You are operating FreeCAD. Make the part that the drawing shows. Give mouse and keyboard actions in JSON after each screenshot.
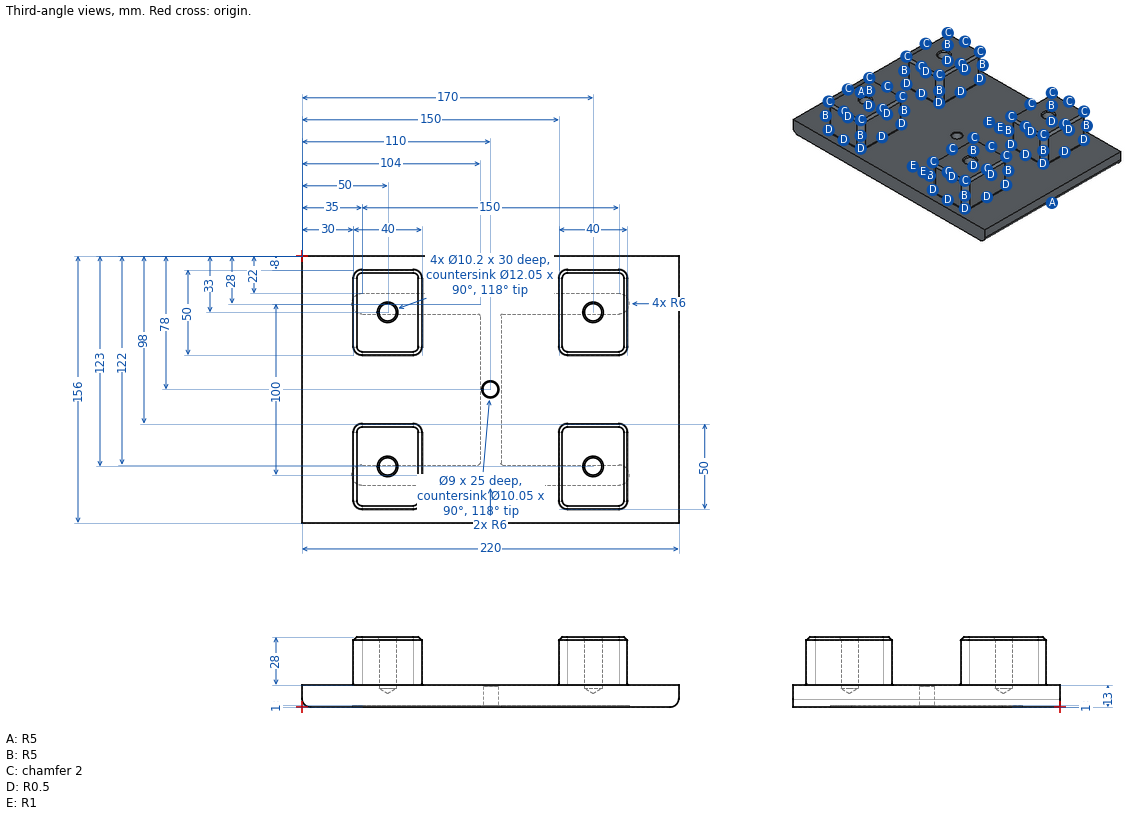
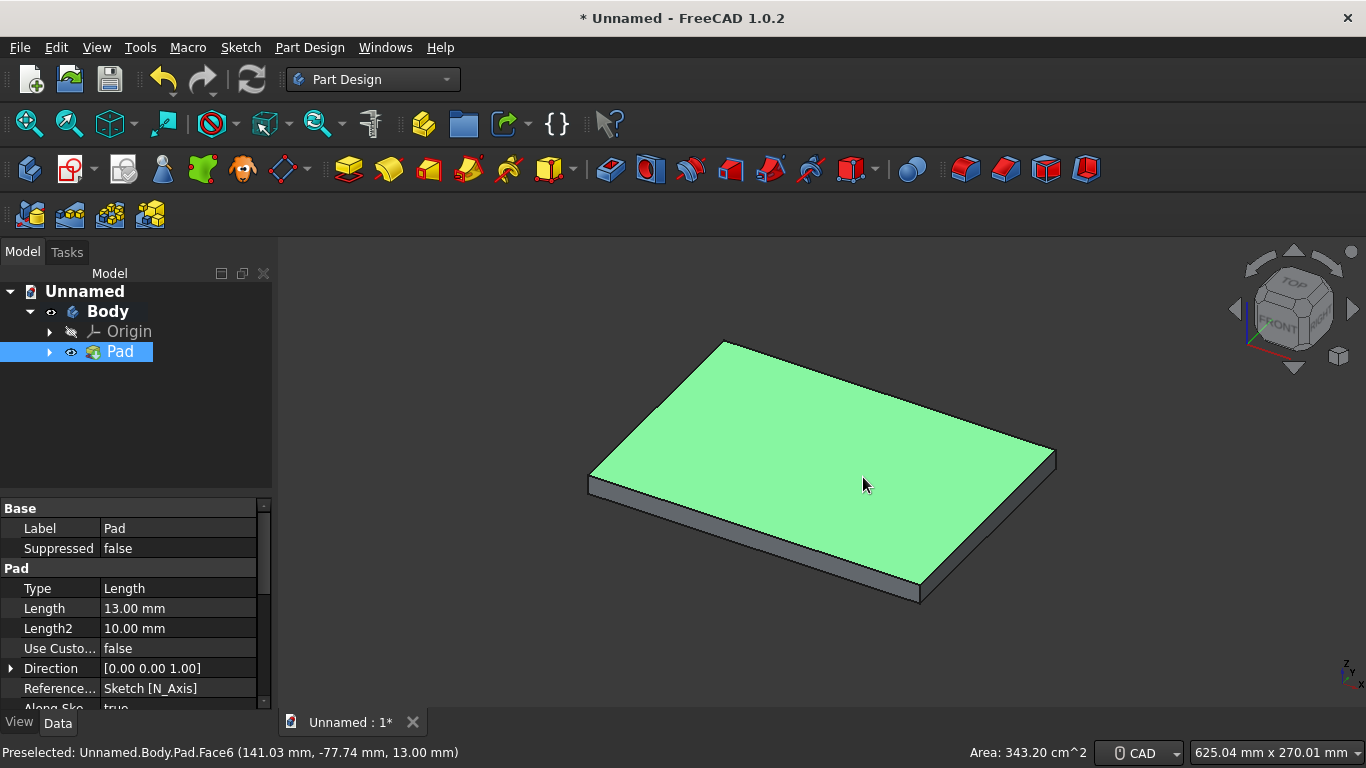
{"action": "left_click", "coordinate": [70, 170]}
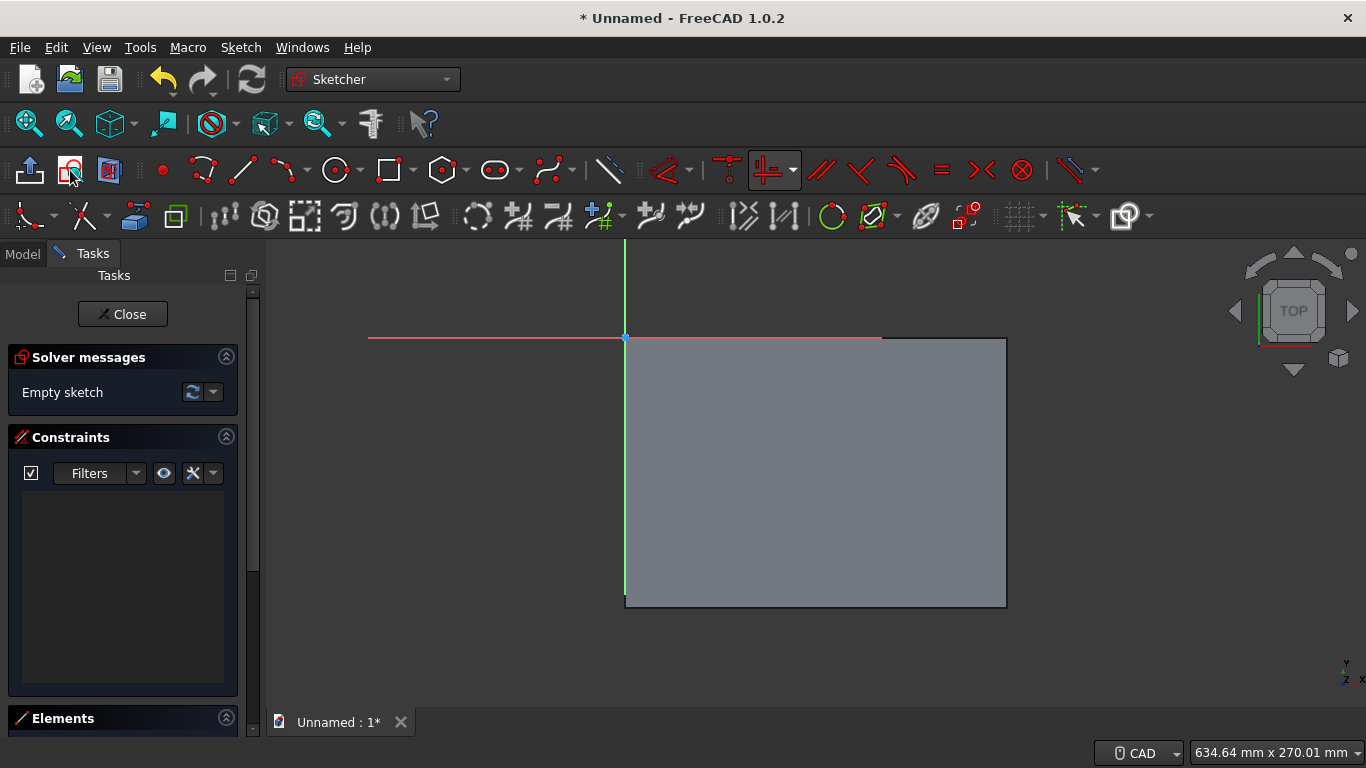
{"action": "key", "text": "g r"}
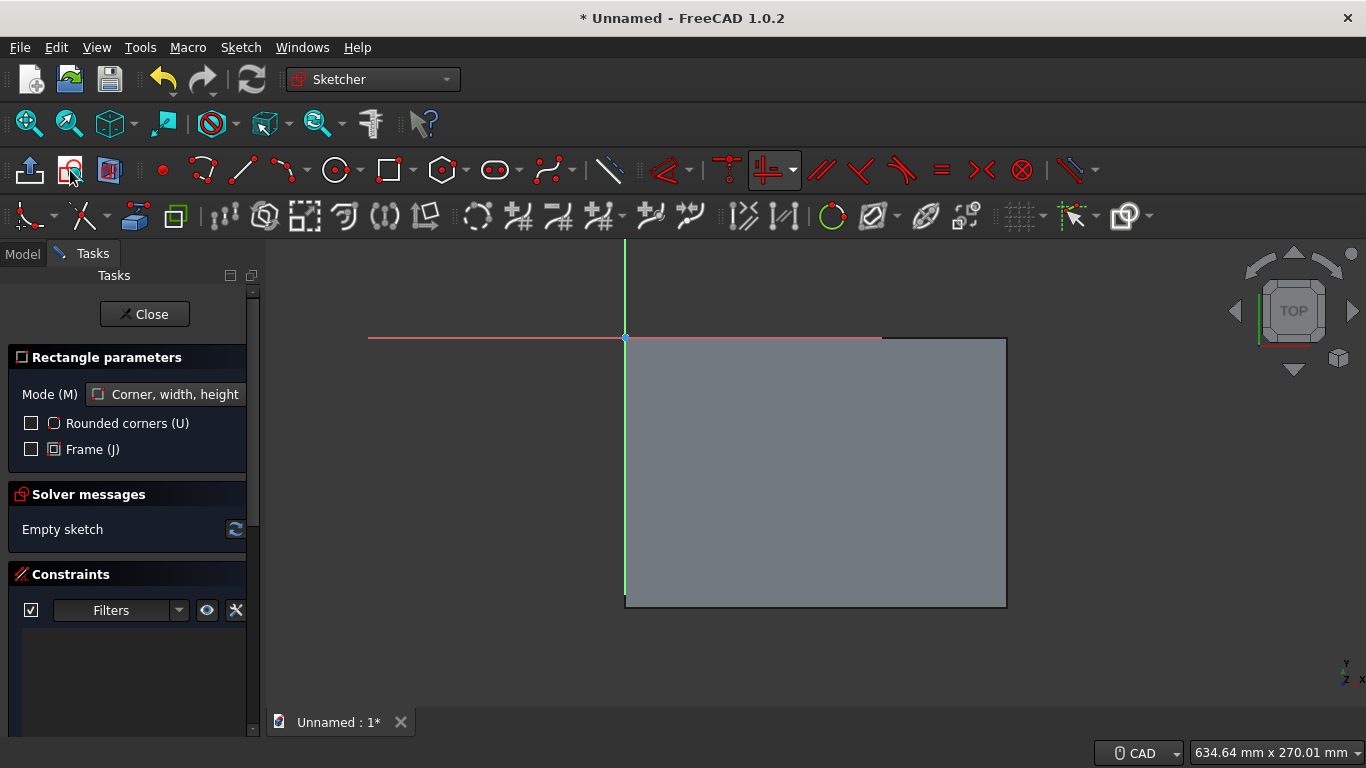
{"action": "left_click", "coordinate": [677, 352]}
{"action": "left_click", "coordinate": [747, 438]}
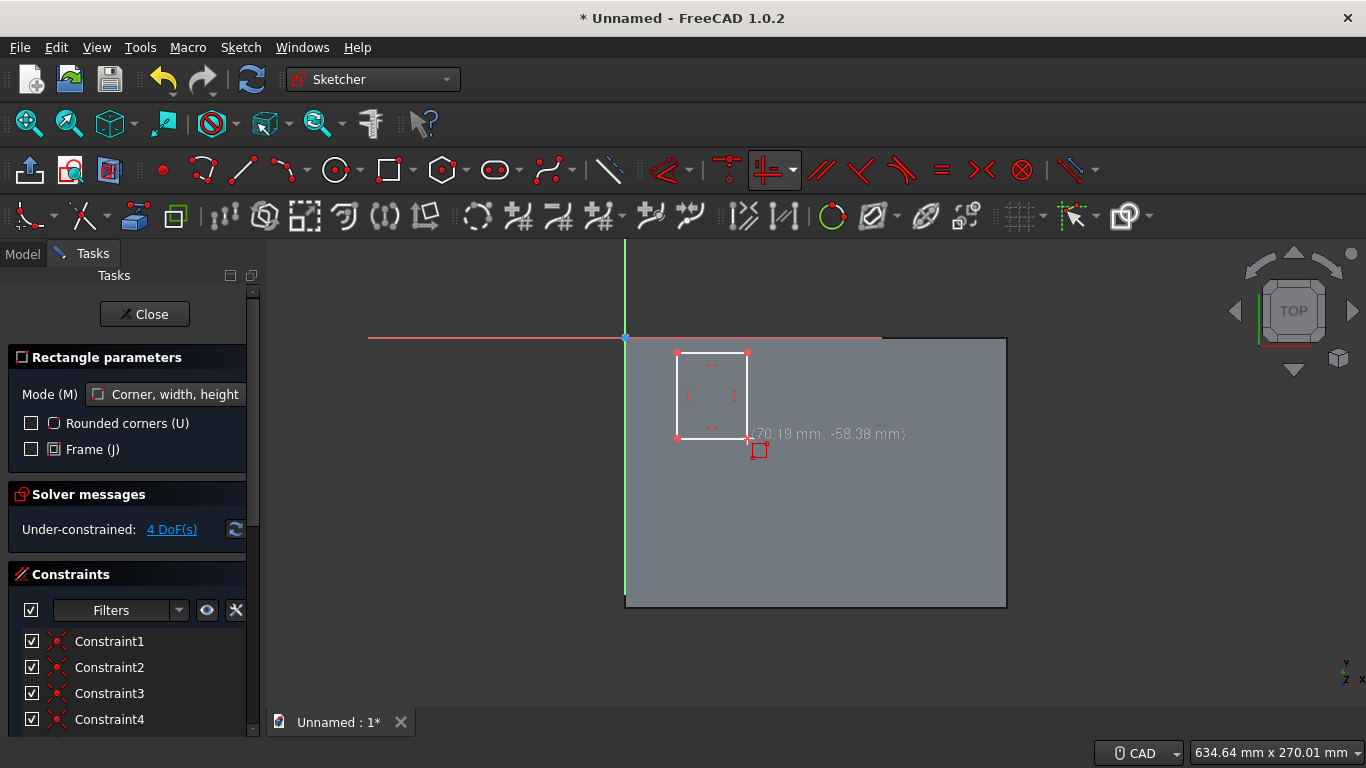
{"action": "left_click", "coordinate": [885, 352]}
{"action": "left_click", "coordinate": [955, 438]}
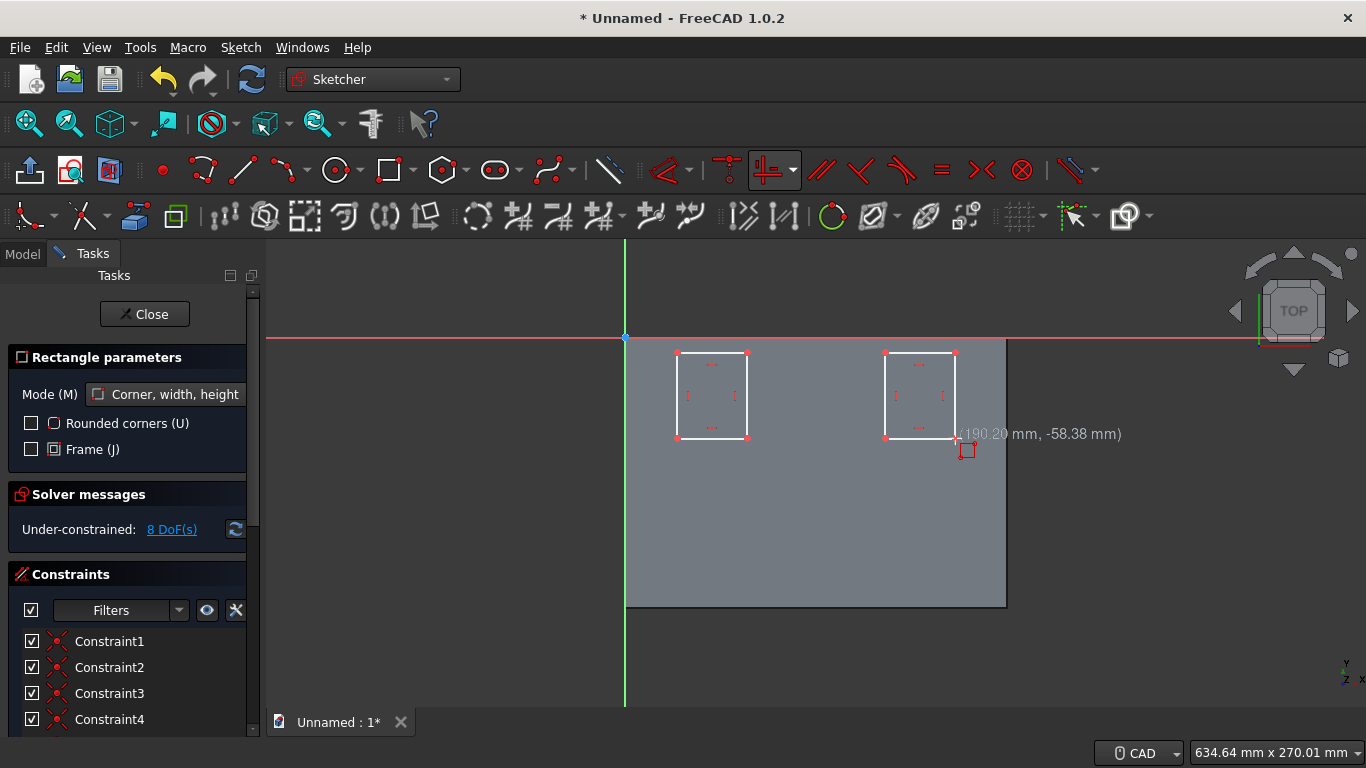
{"action": "left_click", "coordinate": [885, 508]}
{"action": "left_click", "coordinate": [955, 594]}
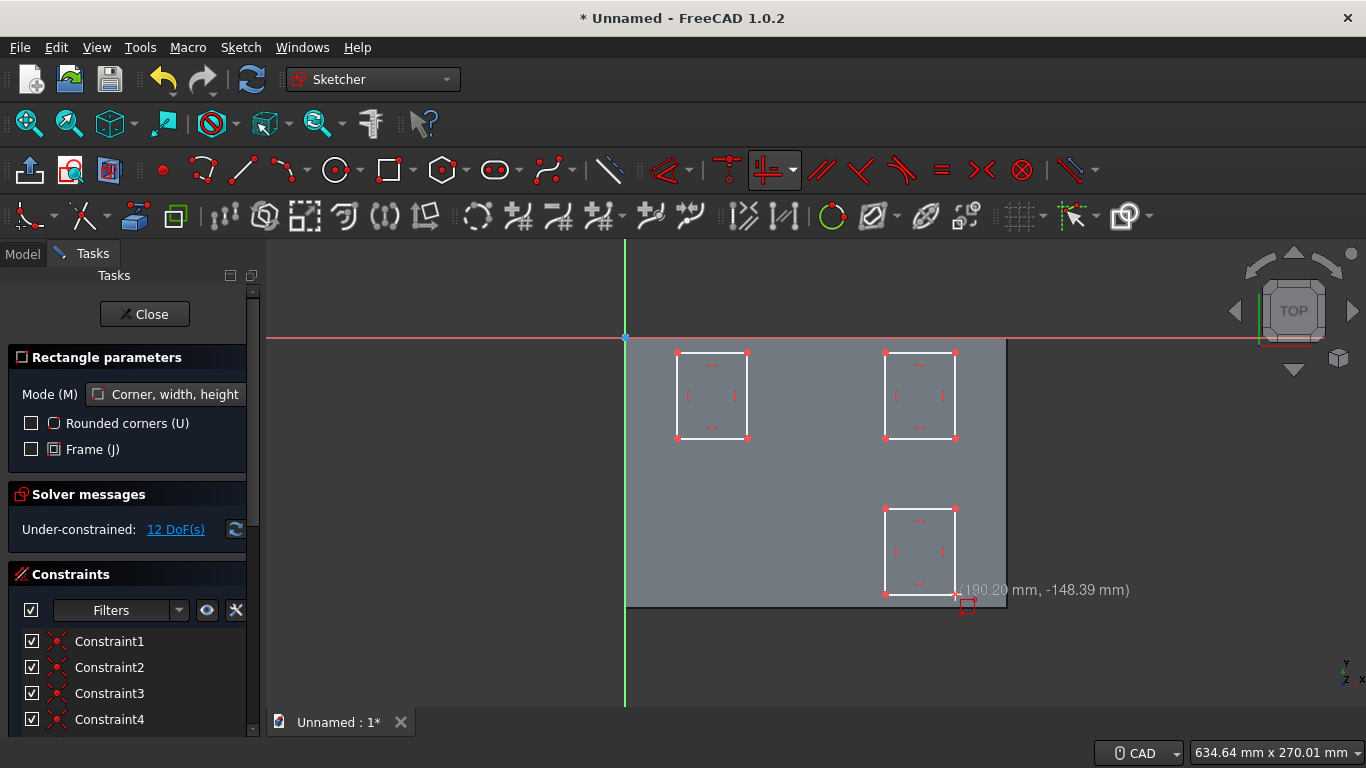
{"action": "left_click", "coordinate": [677, 508]}
{"action": "left_click", "coordinate": [747, 594]}
{"action": "key", "text": "Escape"}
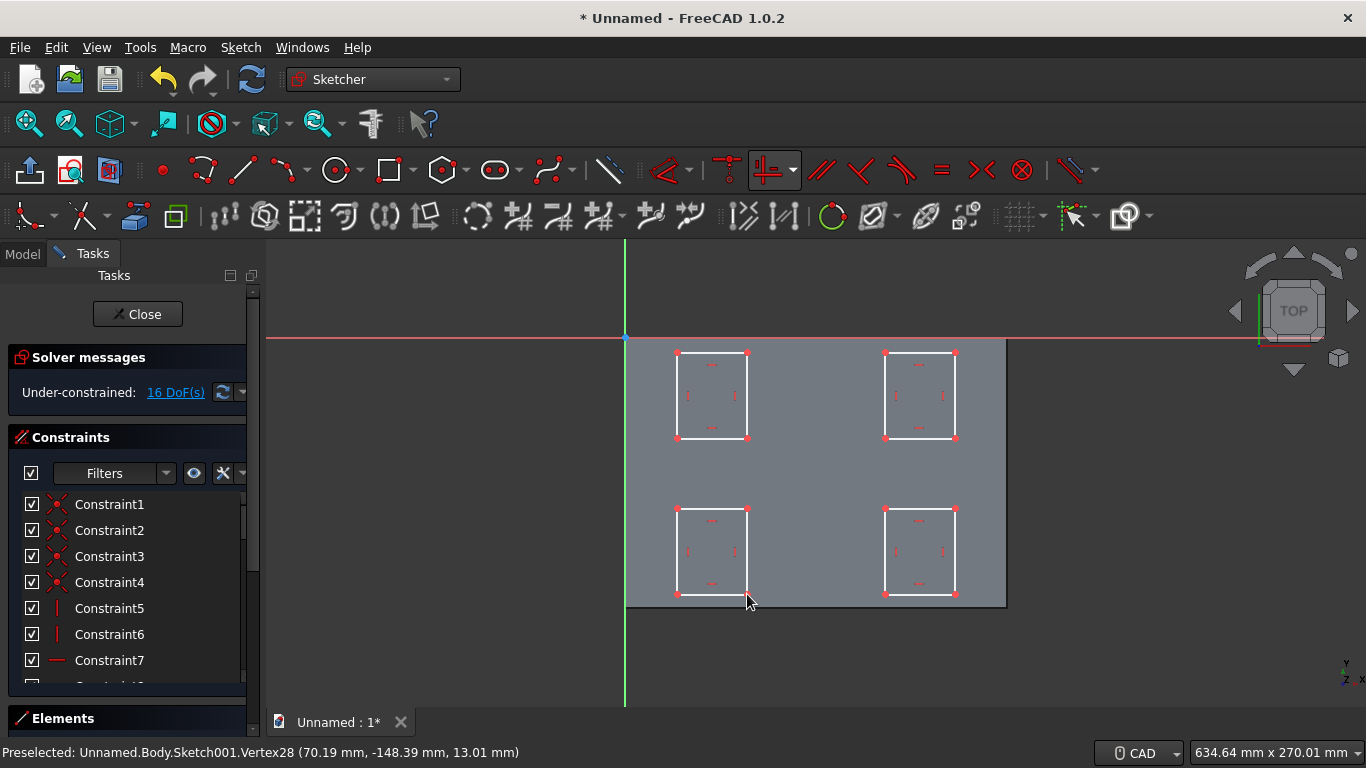
{"action": "key", "text": "d"}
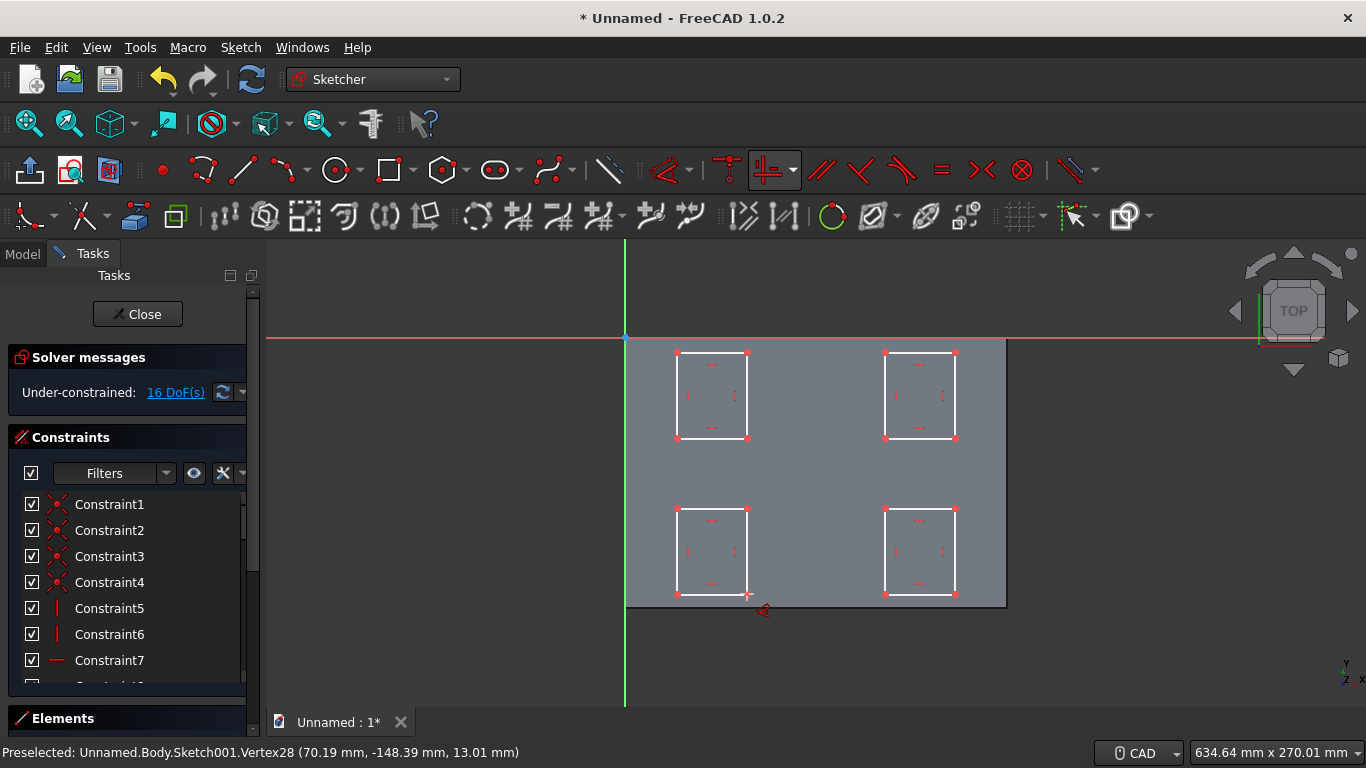
{"action": "left_click", "coordinate": [677, 379]}
{"action": "left_click", "coordinate": [643, 396]}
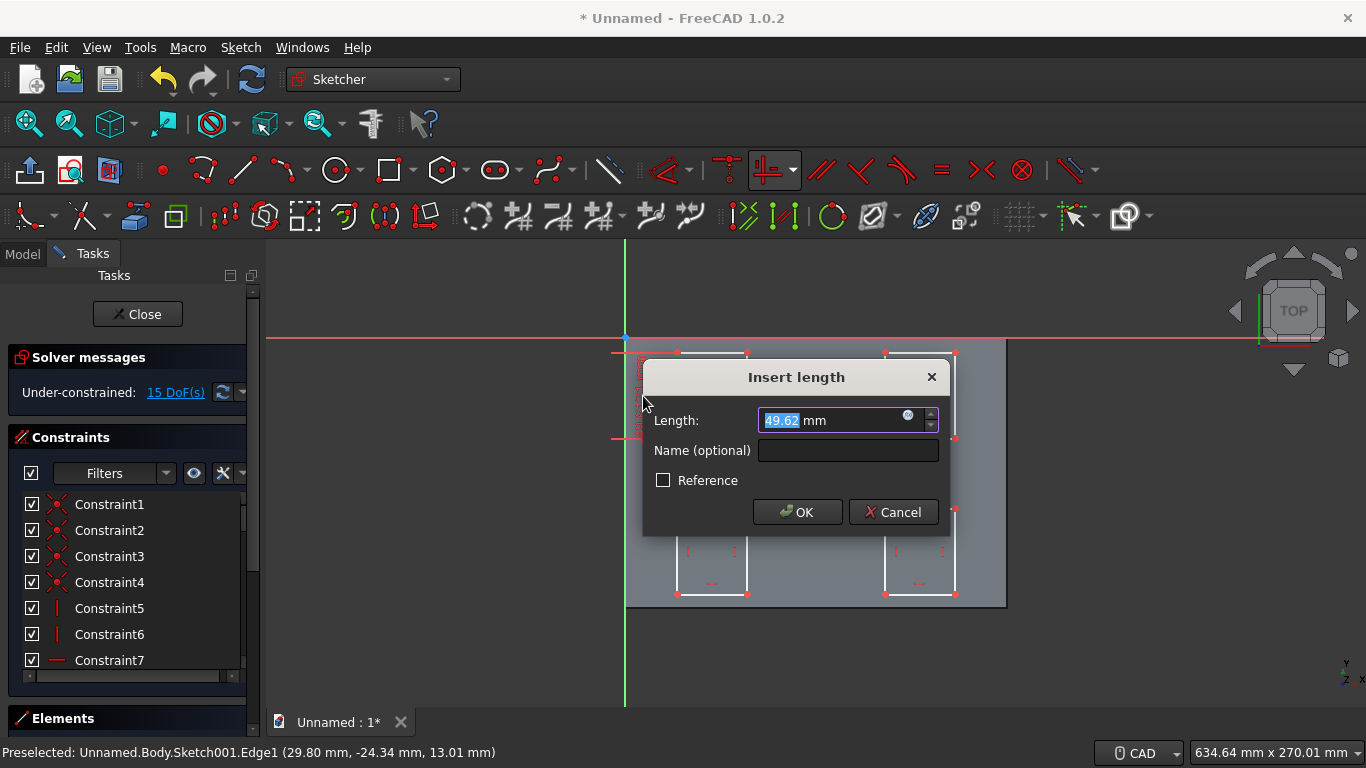
{"action": "type", "text": "50"}
{"action": "key", "text": "Return"}